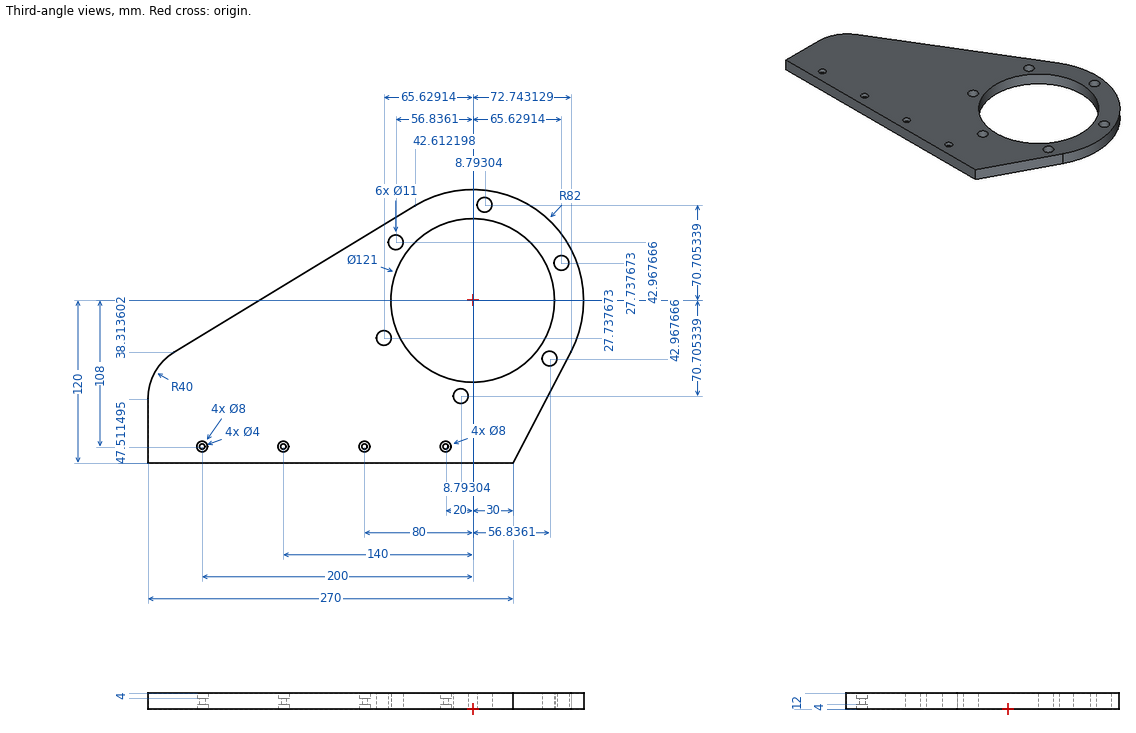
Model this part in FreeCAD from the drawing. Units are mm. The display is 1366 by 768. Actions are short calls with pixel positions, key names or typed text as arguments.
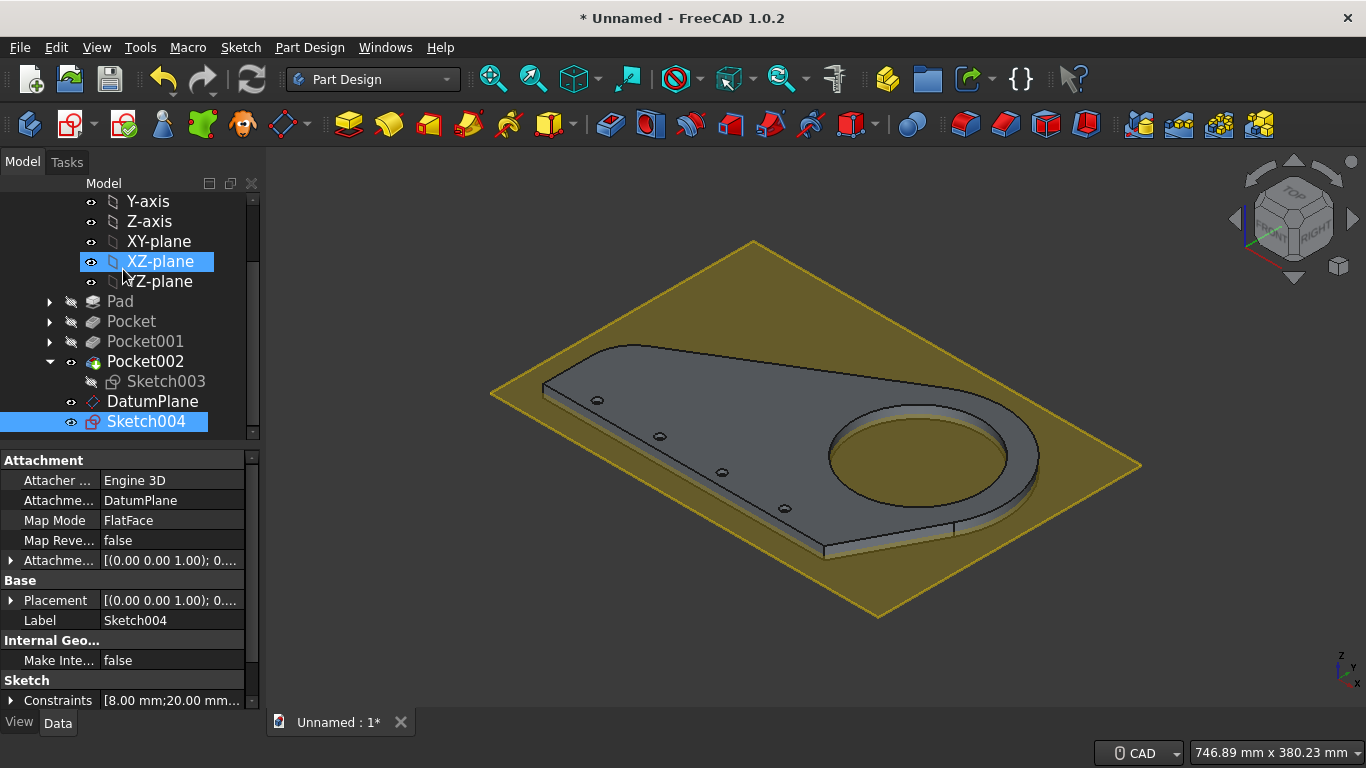
click(612, 124)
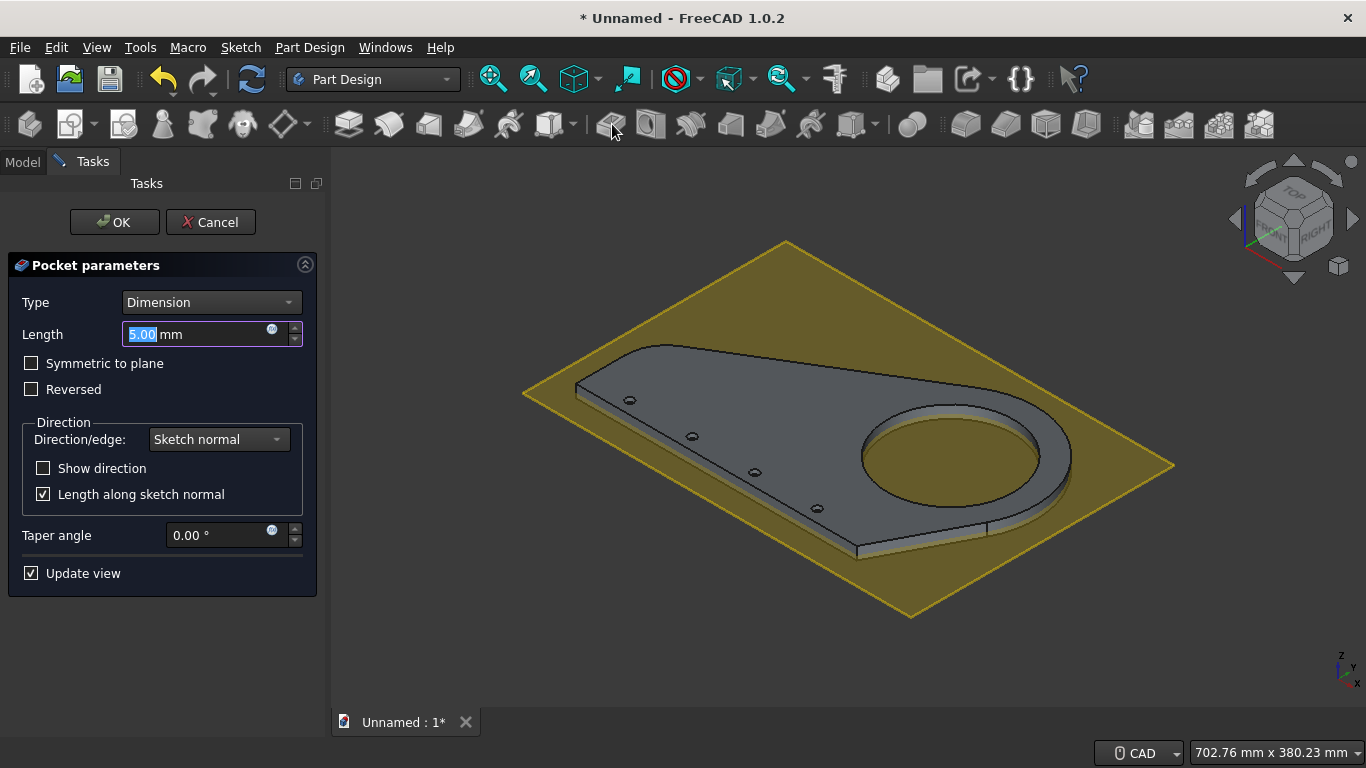
text(4)
key(Tab)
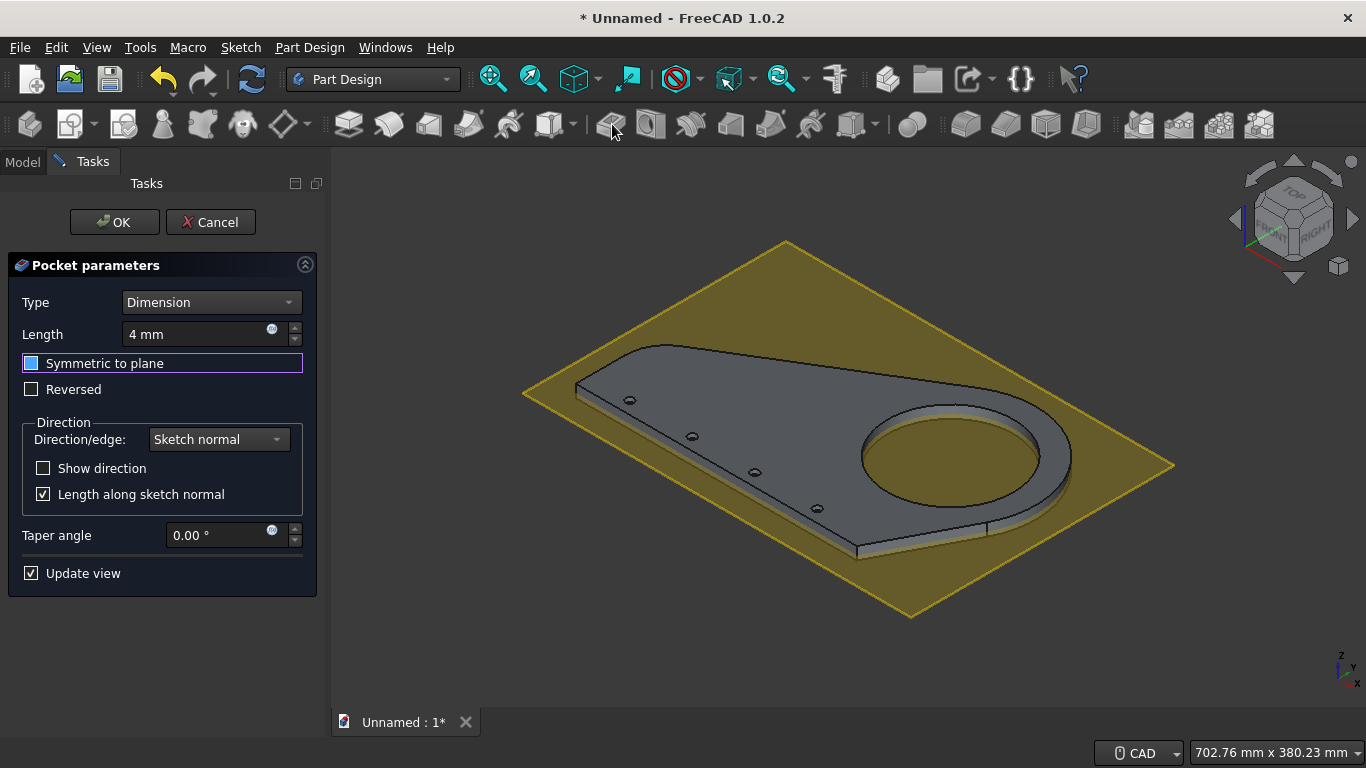
click(115, 222)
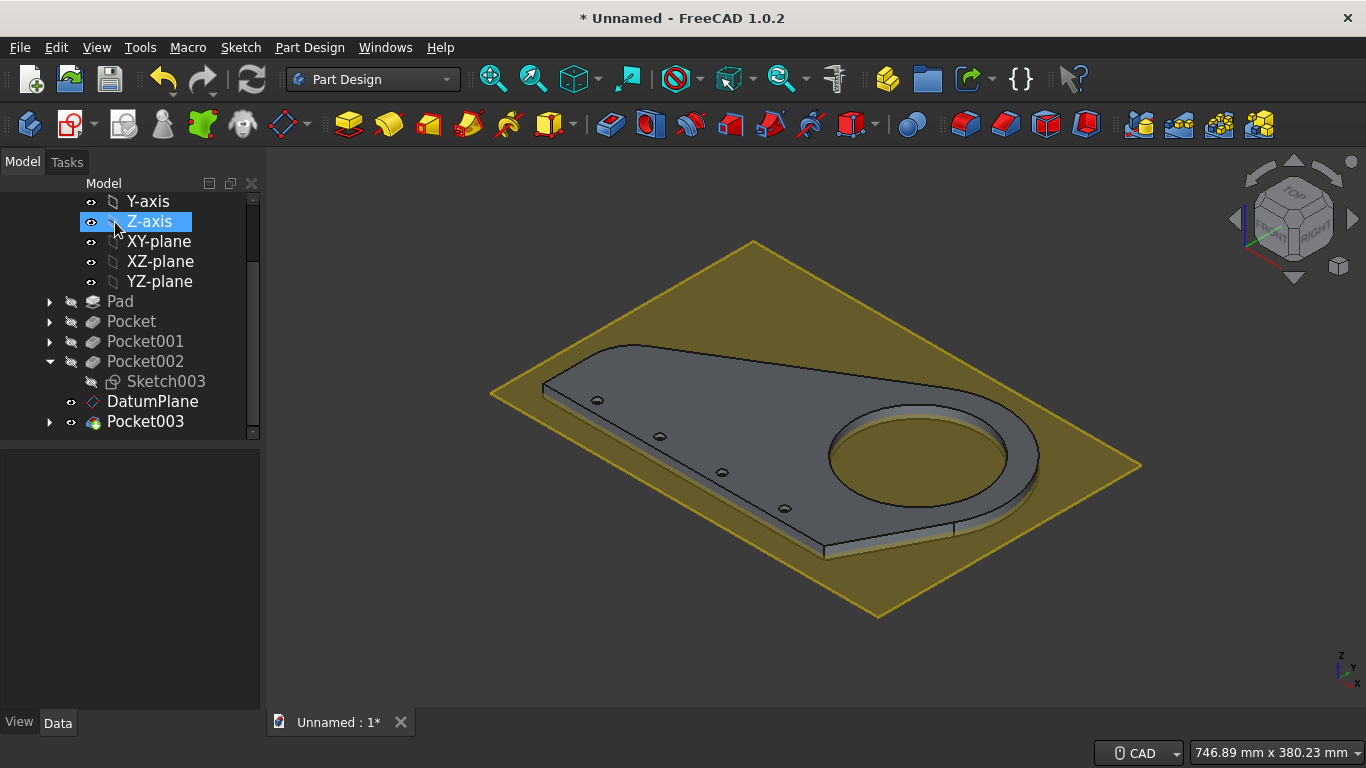
click(116, 402)
key(space)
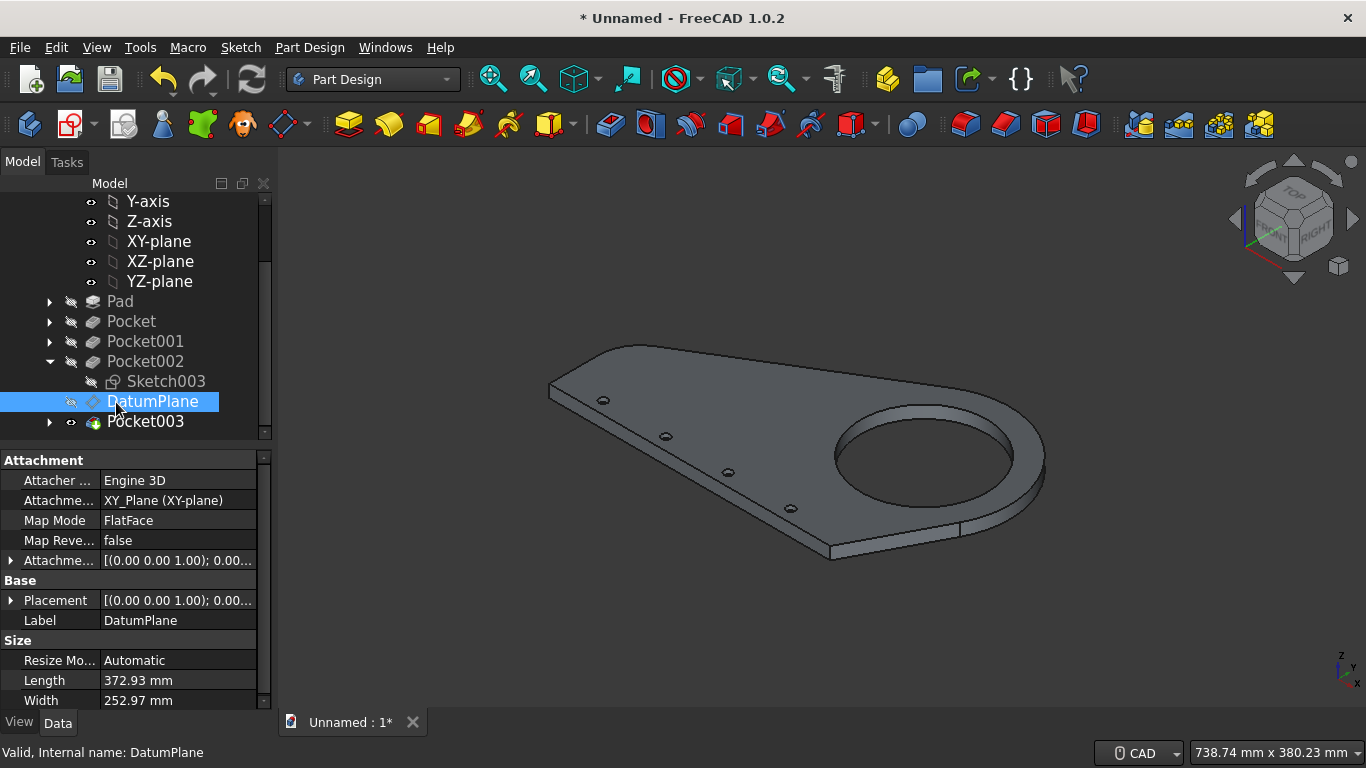
key(5)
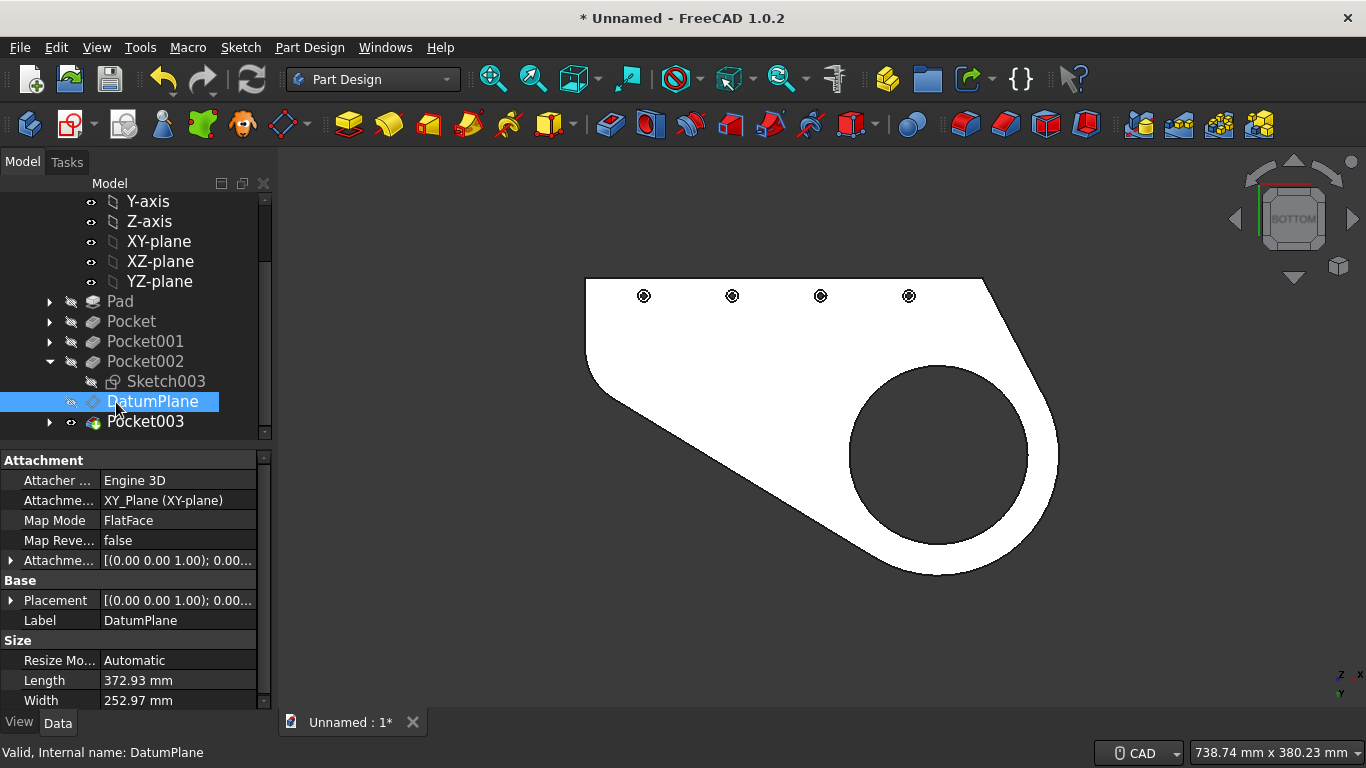
click(754, 384)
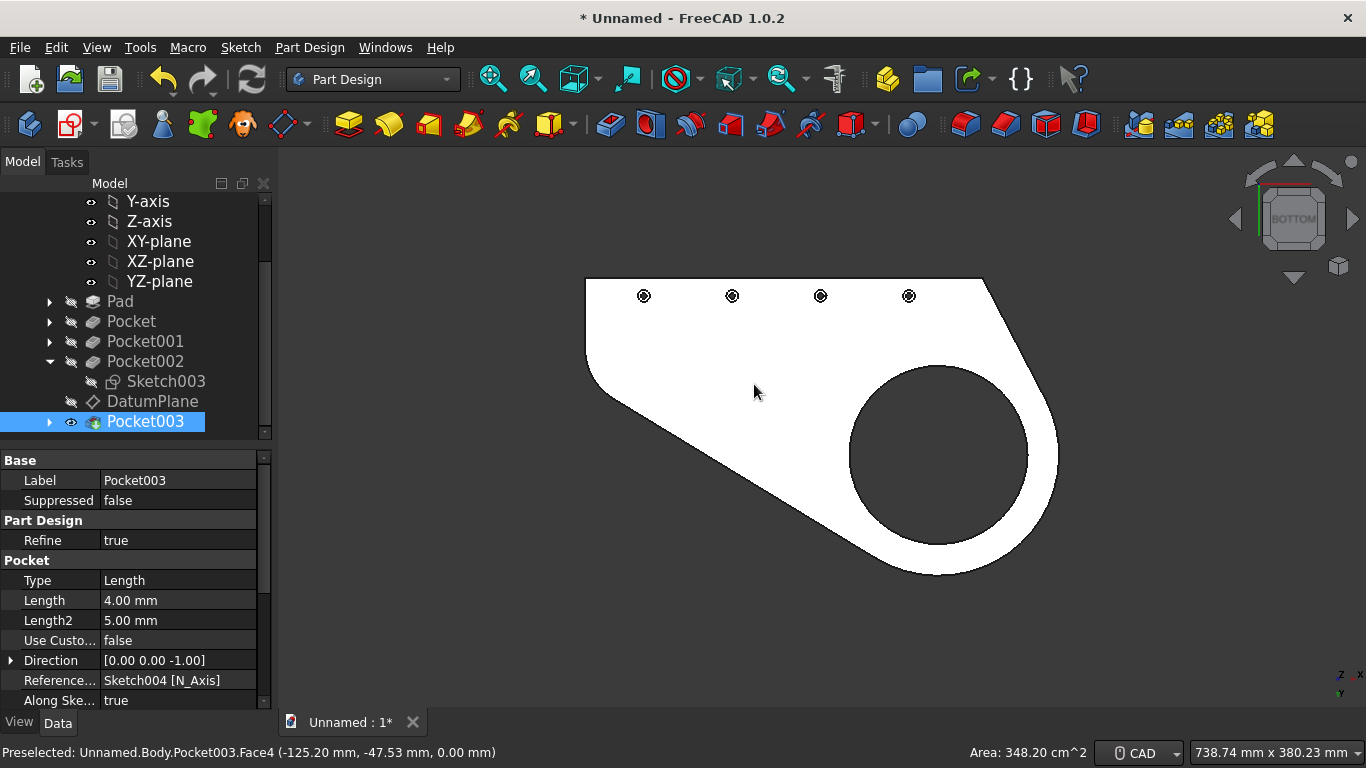
click(70, 124)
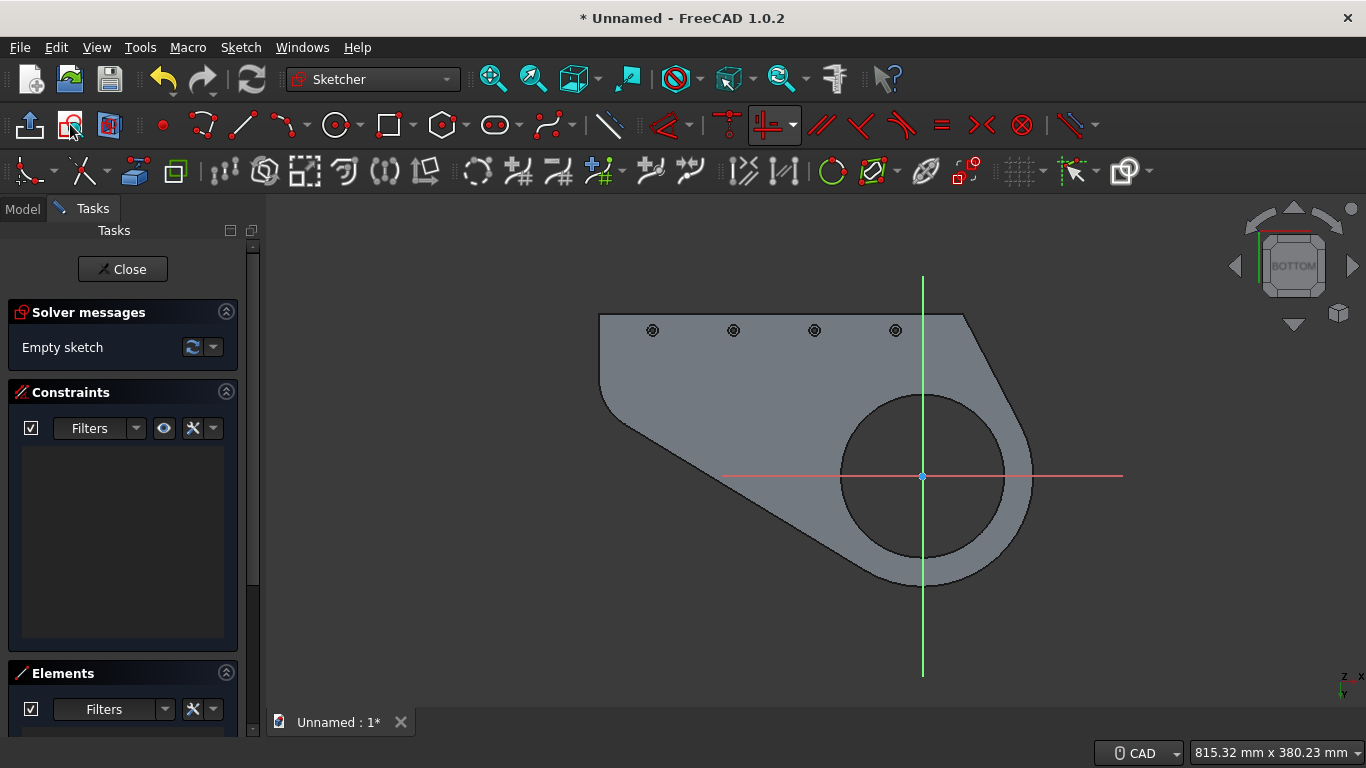
scroll(1201, 528, up, 2)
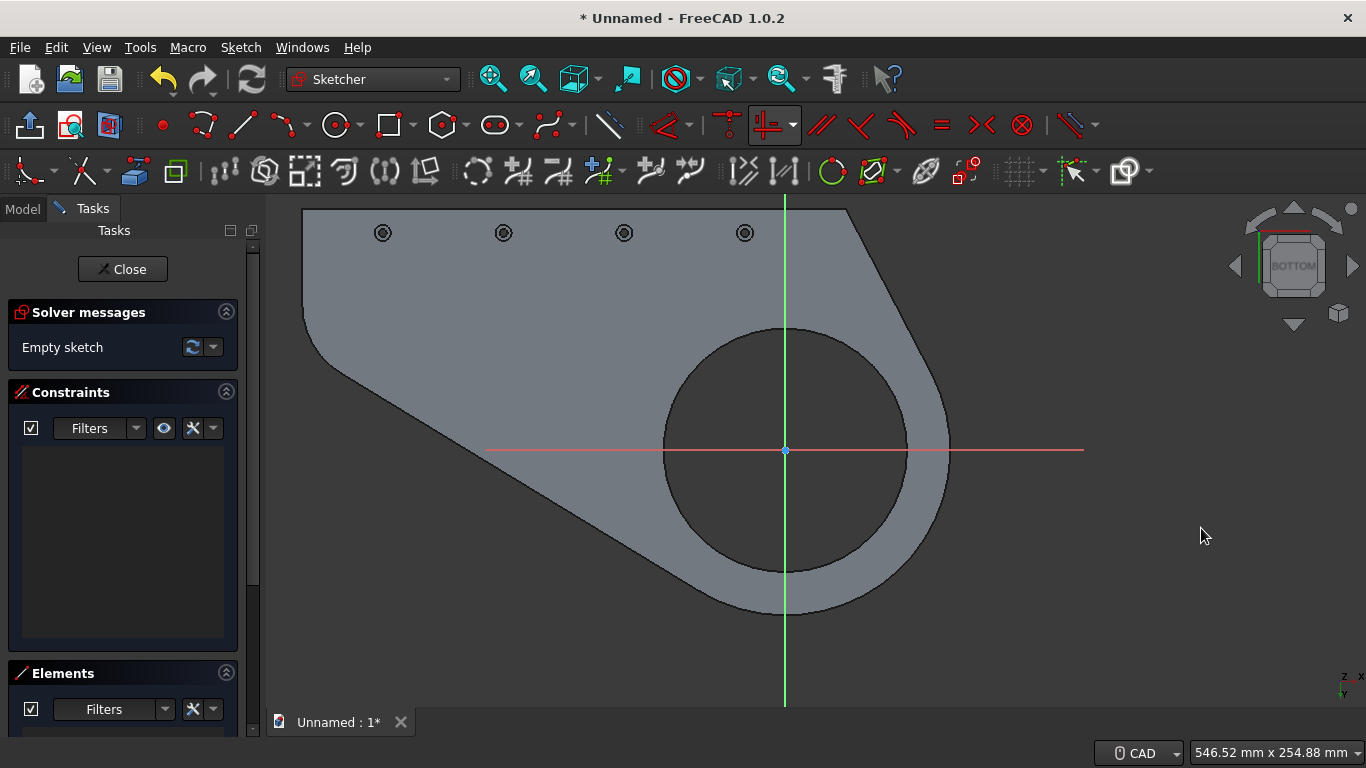
click(336, 126)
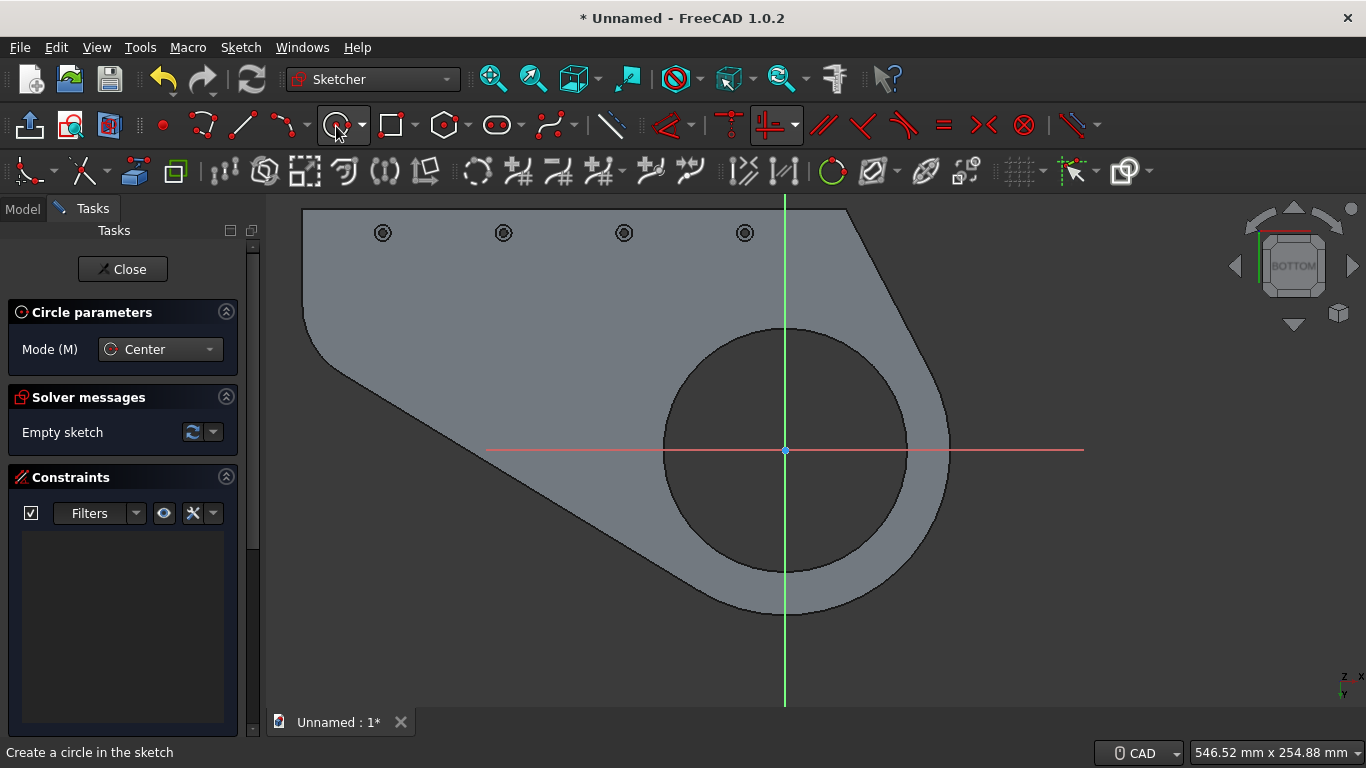
scroll(671, 537, up, 4)